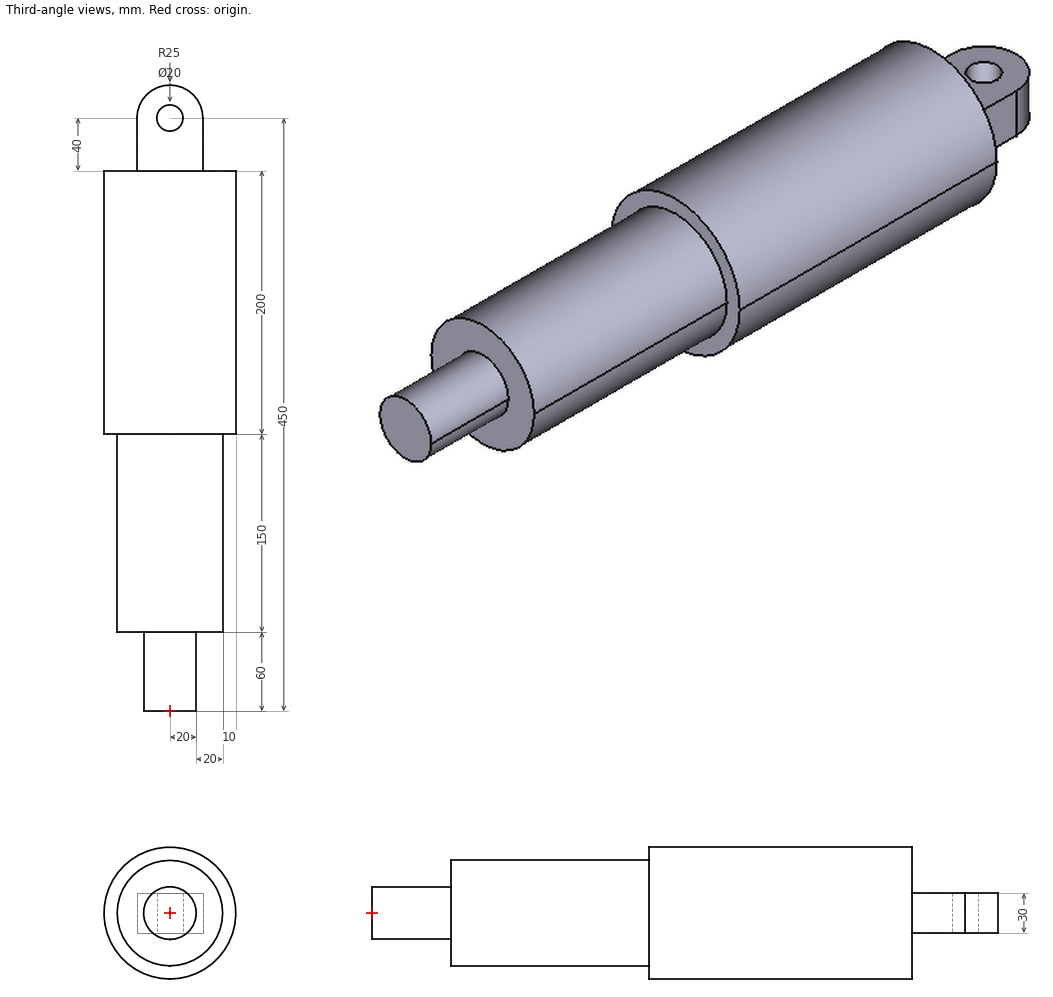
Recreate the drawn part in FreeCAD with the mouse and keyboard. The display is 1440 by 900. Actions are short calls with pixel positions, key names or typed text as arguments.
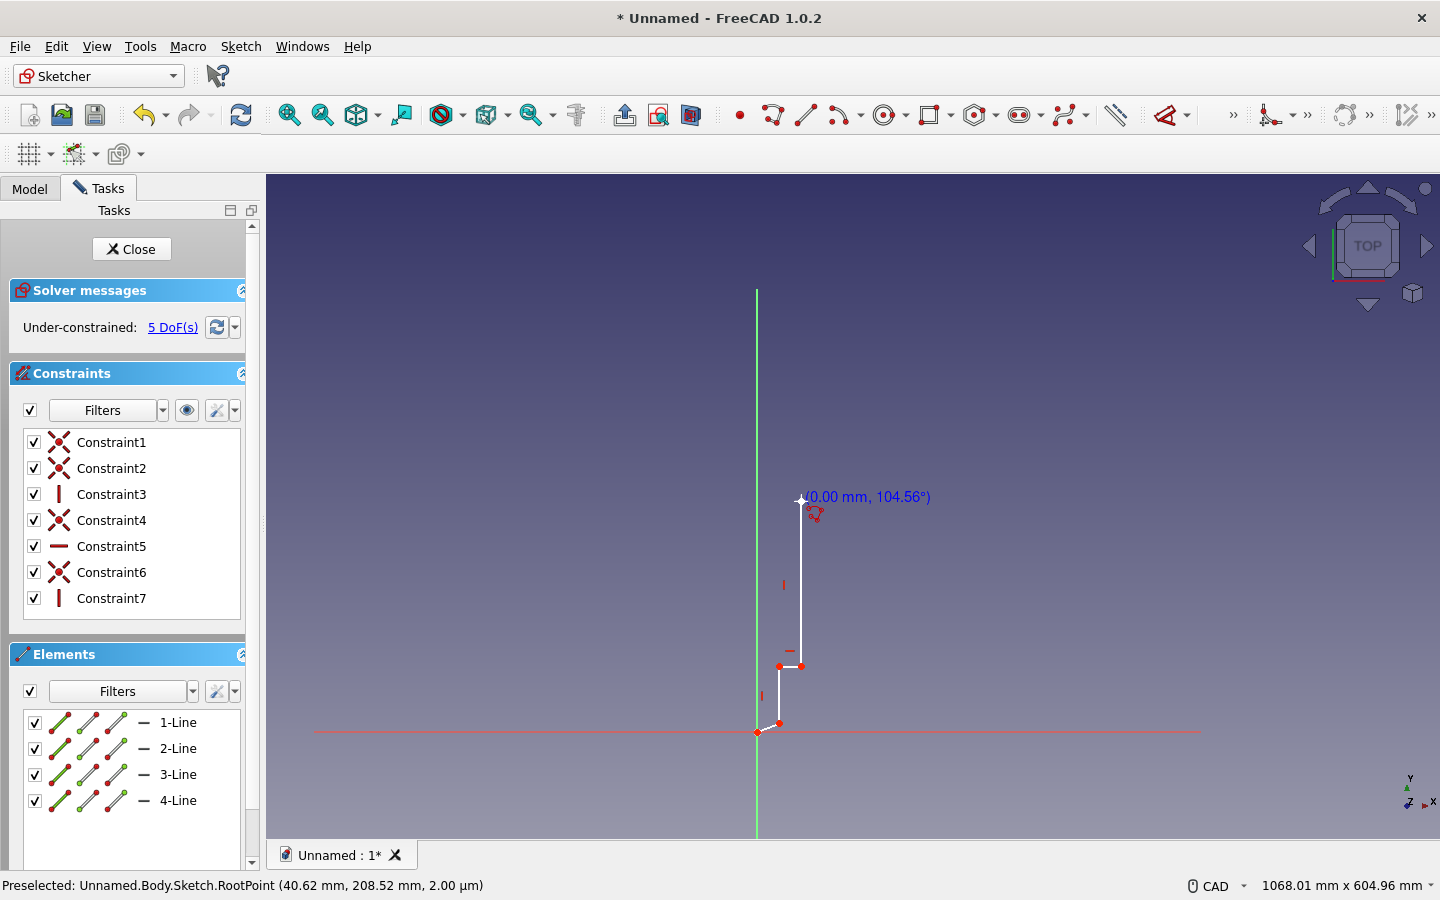
scroll(812, 501, up, 2)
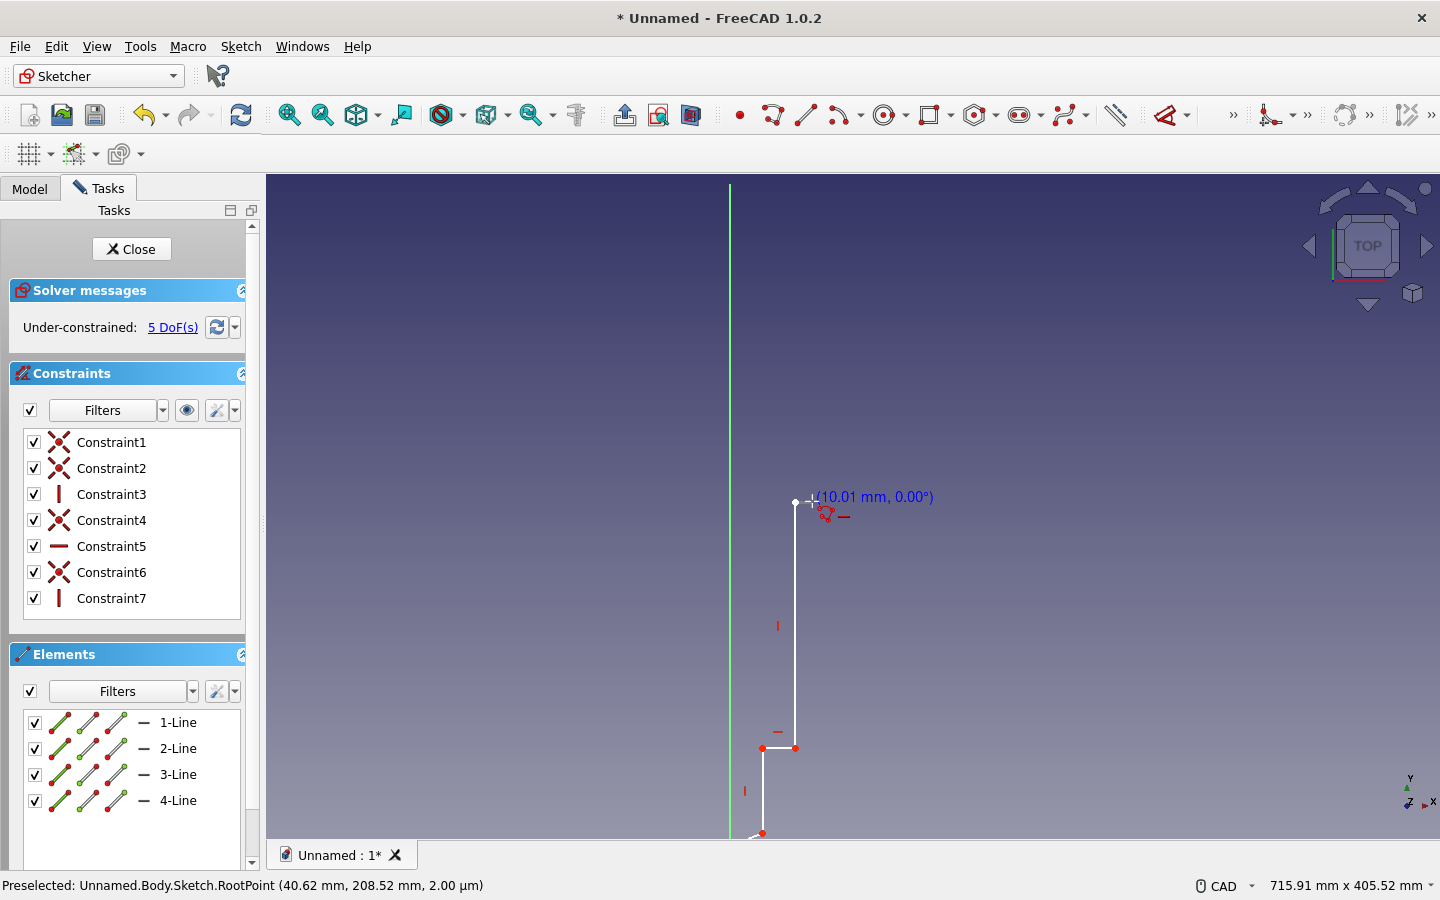
click(812, 501)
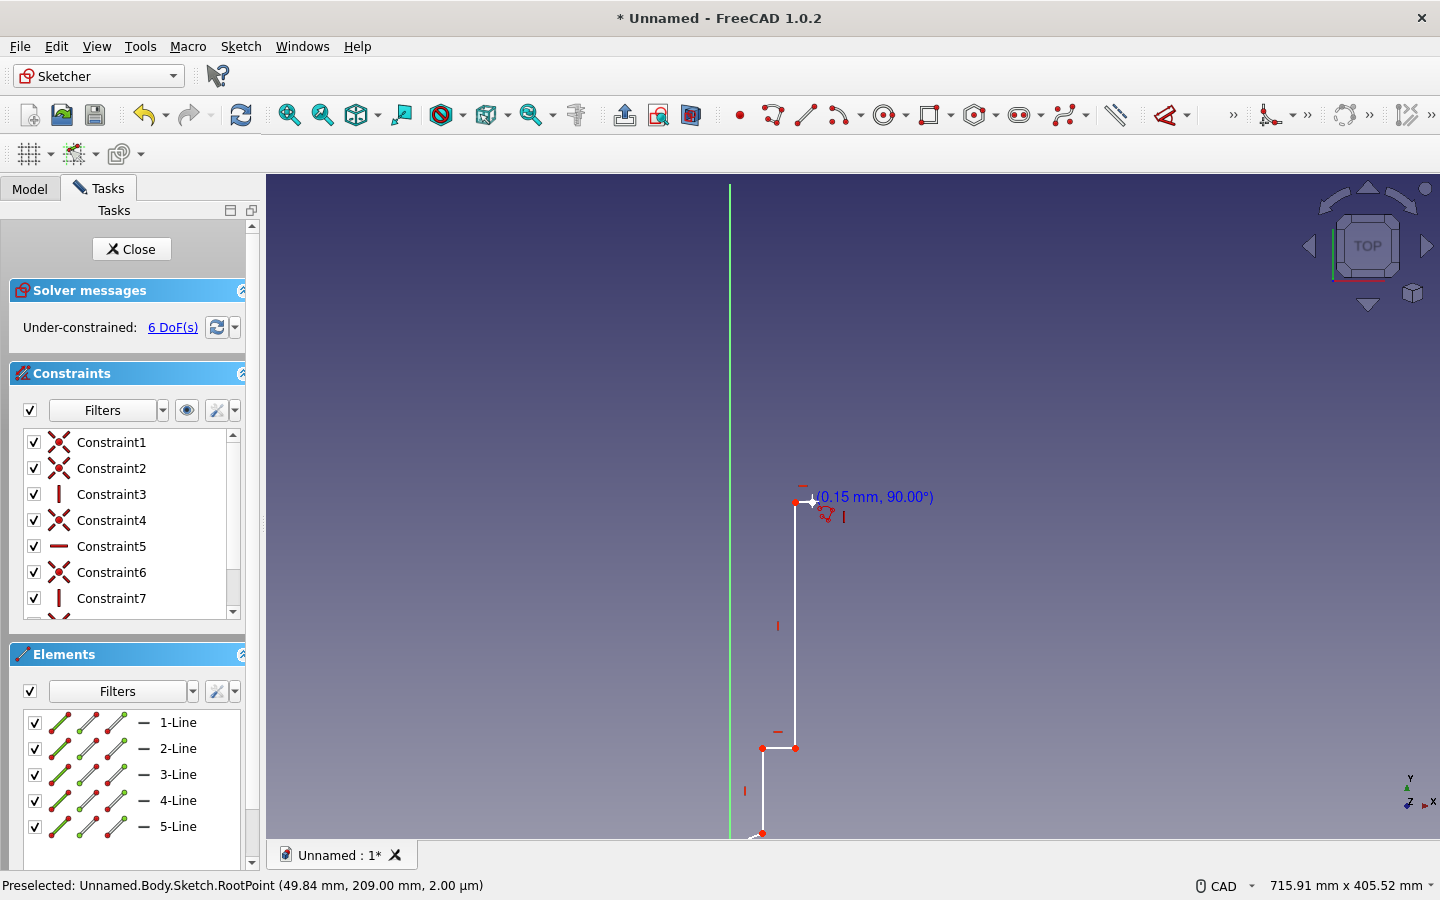
scroll(811, 500, down, 2)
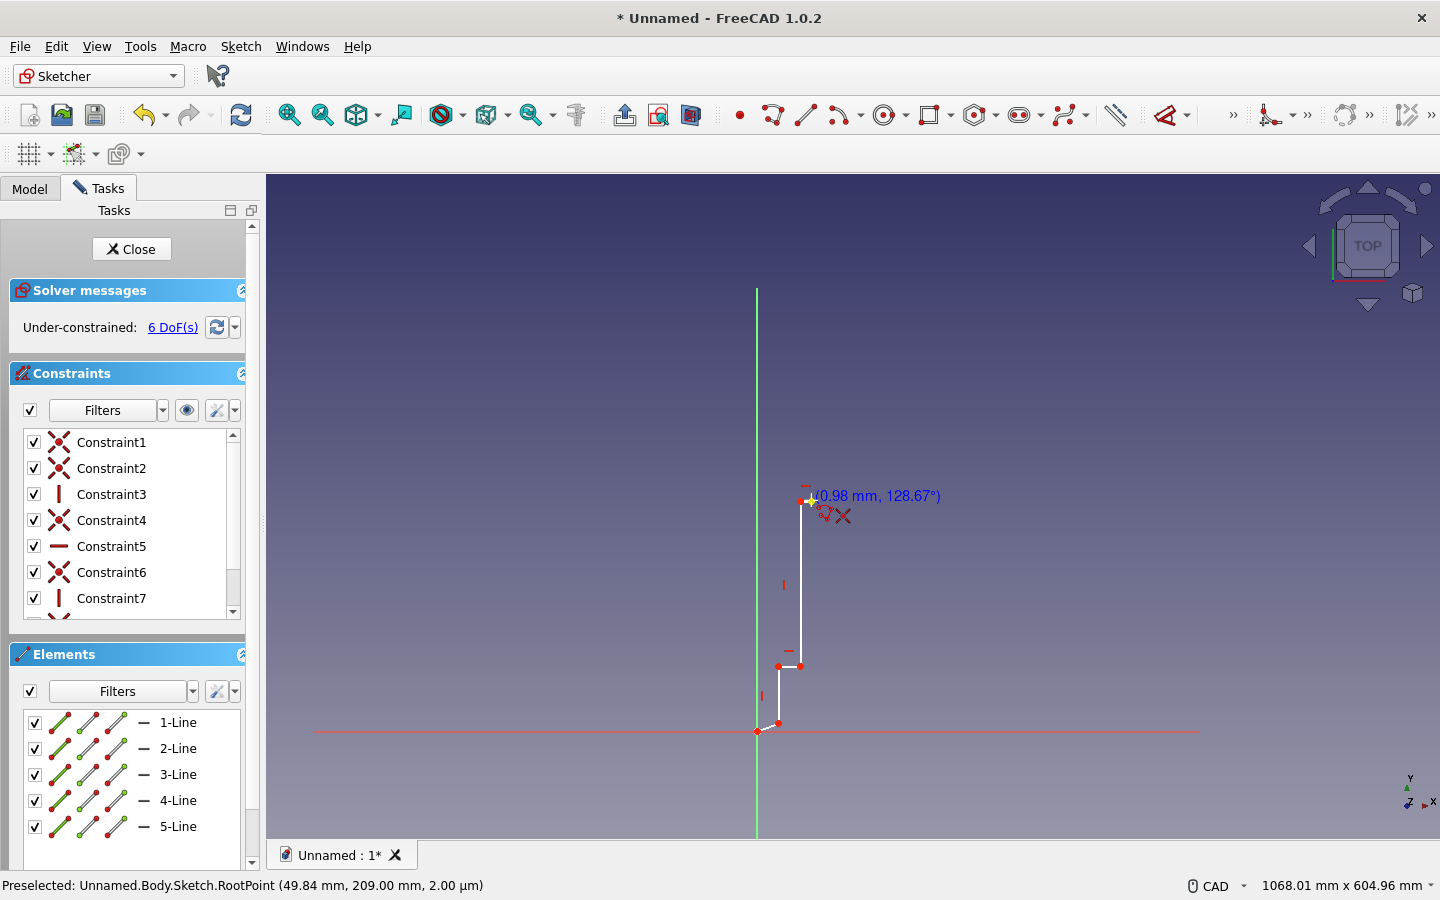
click(812, 281)
click(766, 281)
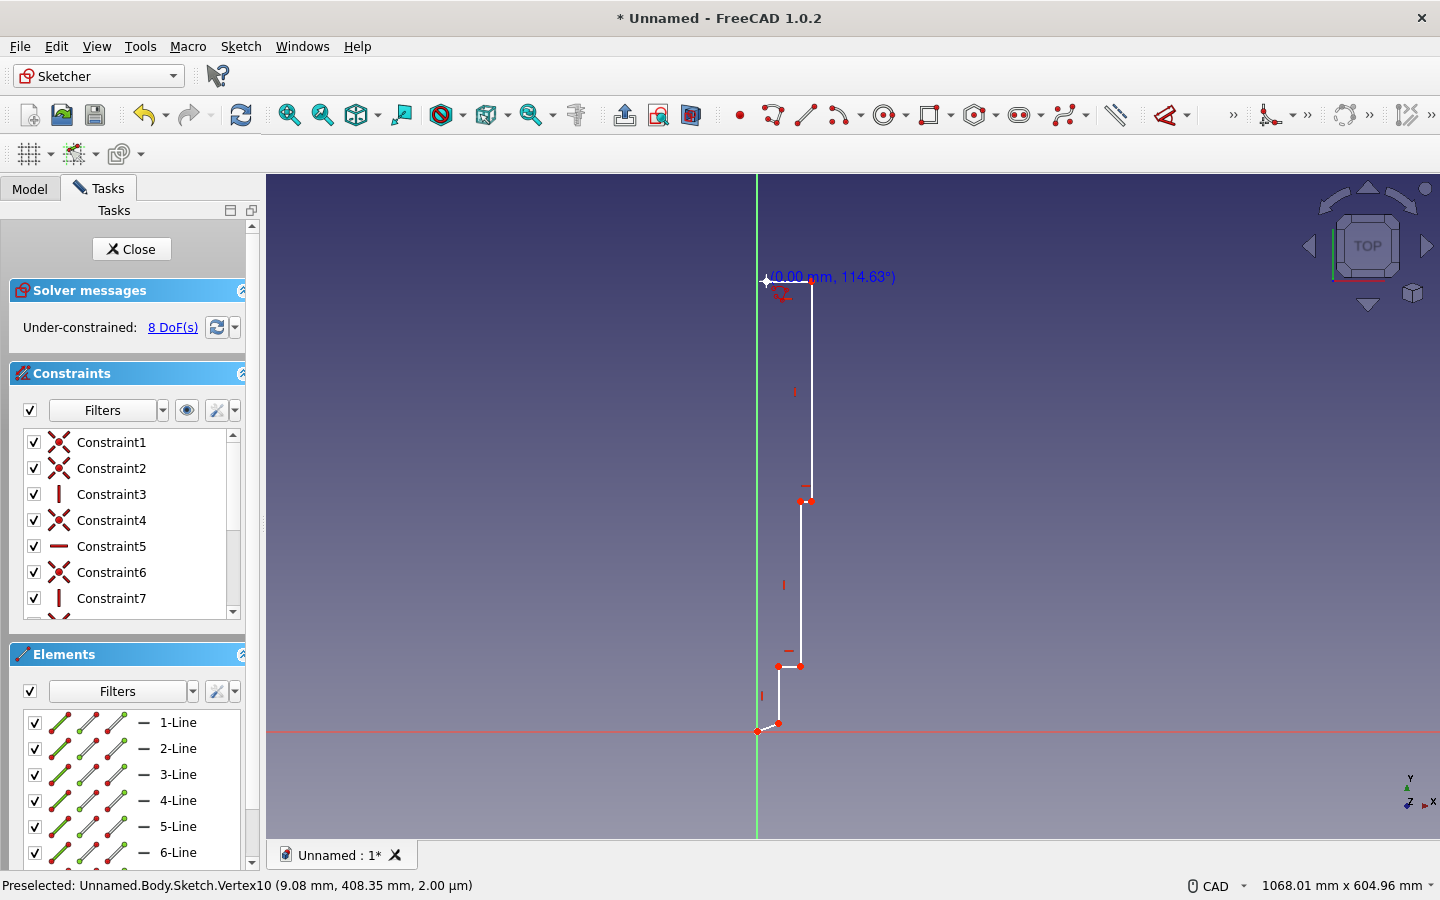
scroll(757, 732, up, 2)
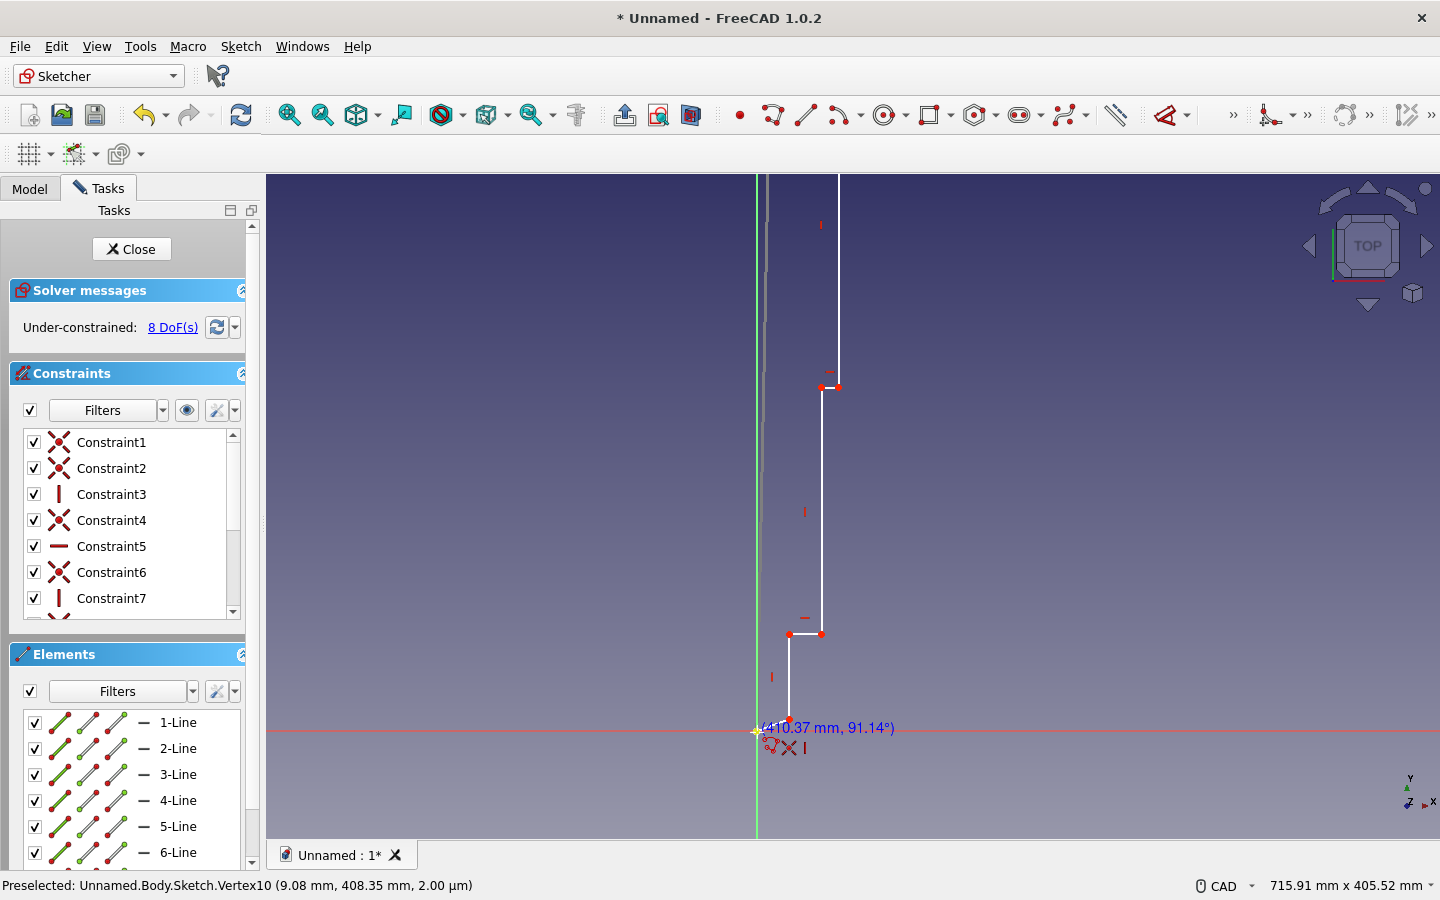
click(757, 731)
key(Escape)
key(Escape)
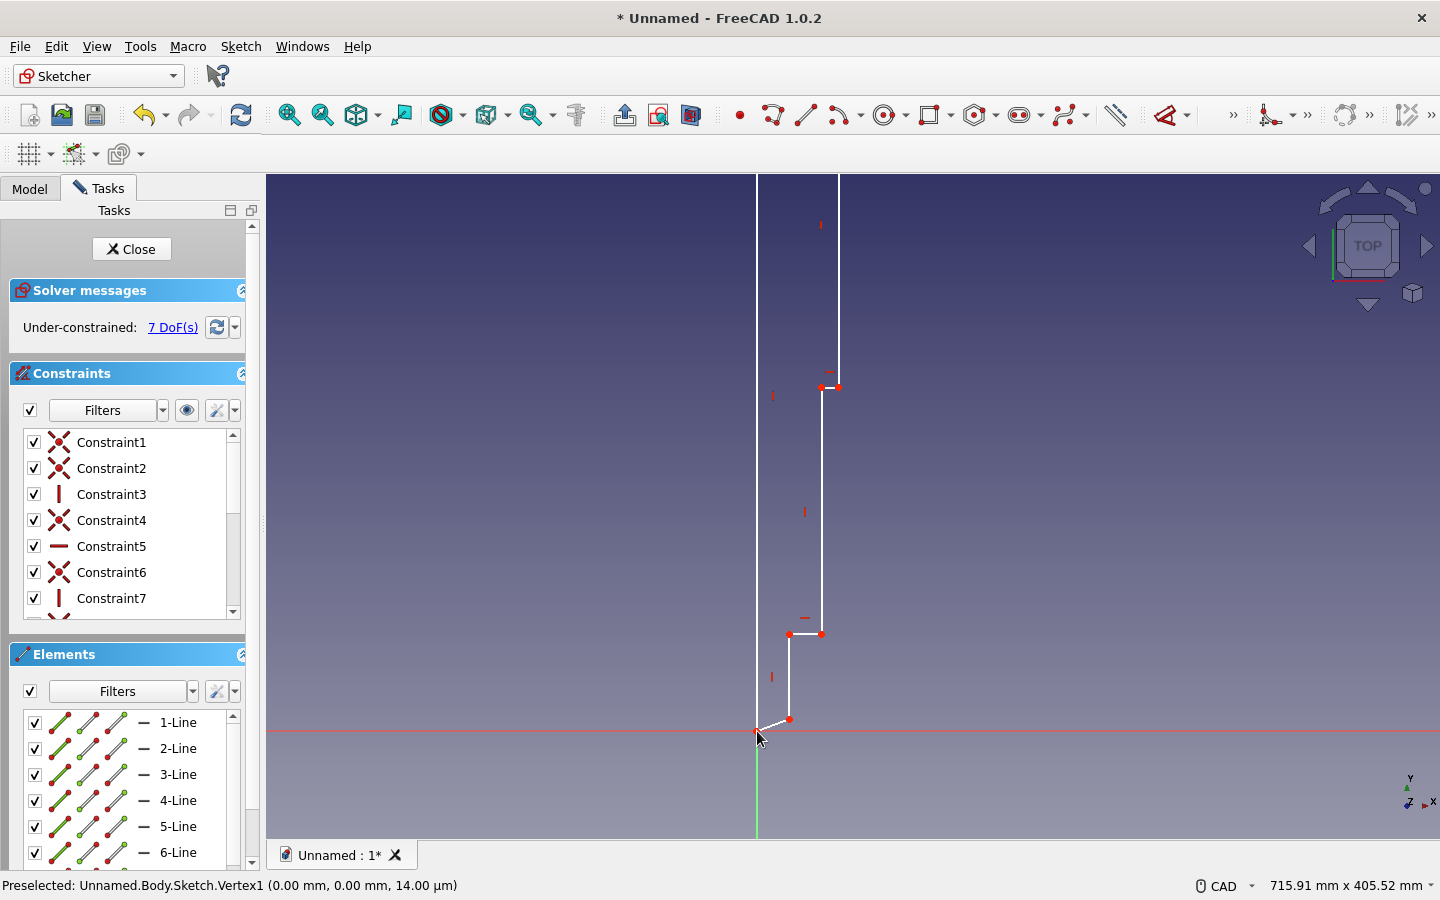
scroll(767, 728, up, 2)